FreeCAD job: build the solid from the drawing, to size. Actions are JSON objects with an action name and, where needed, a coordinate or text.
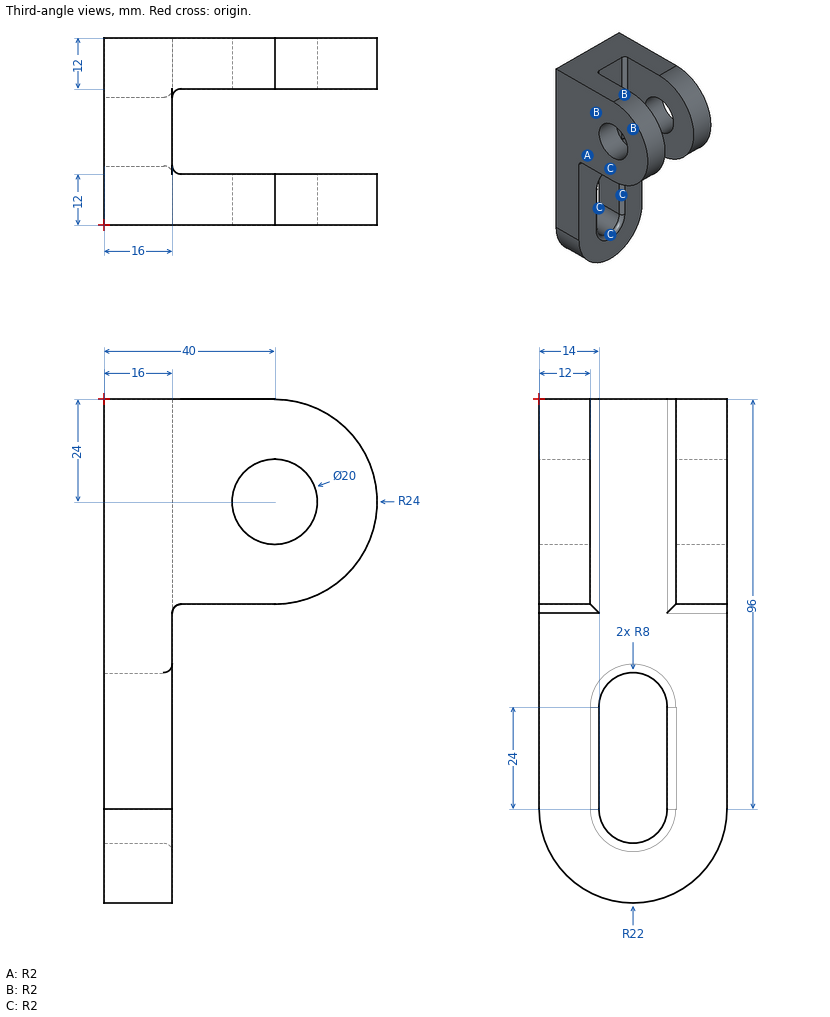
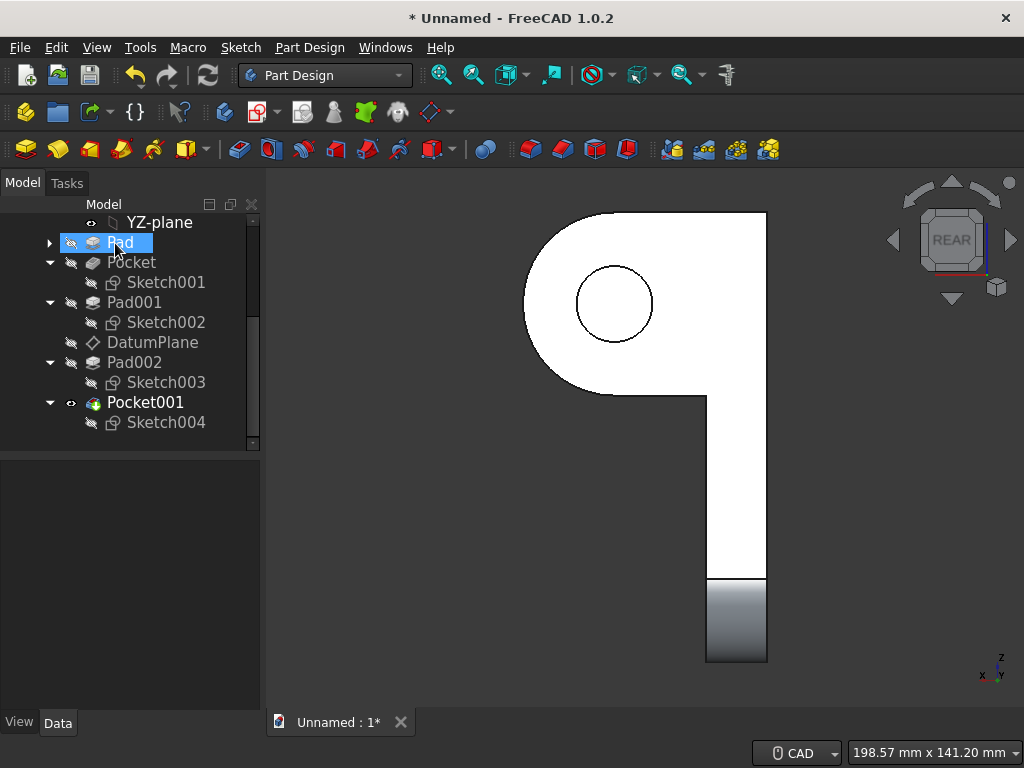
{"action": "left_click", "coordinate": [614, 303]}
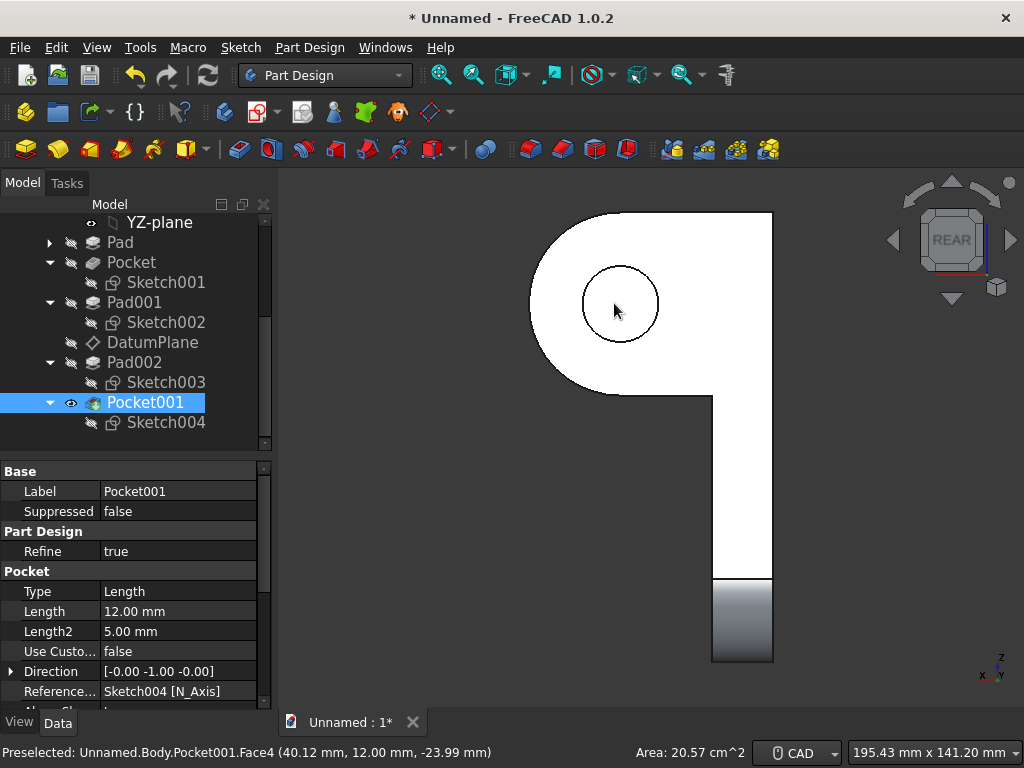
{"action": "left_click", "coordinate": [258, 112]}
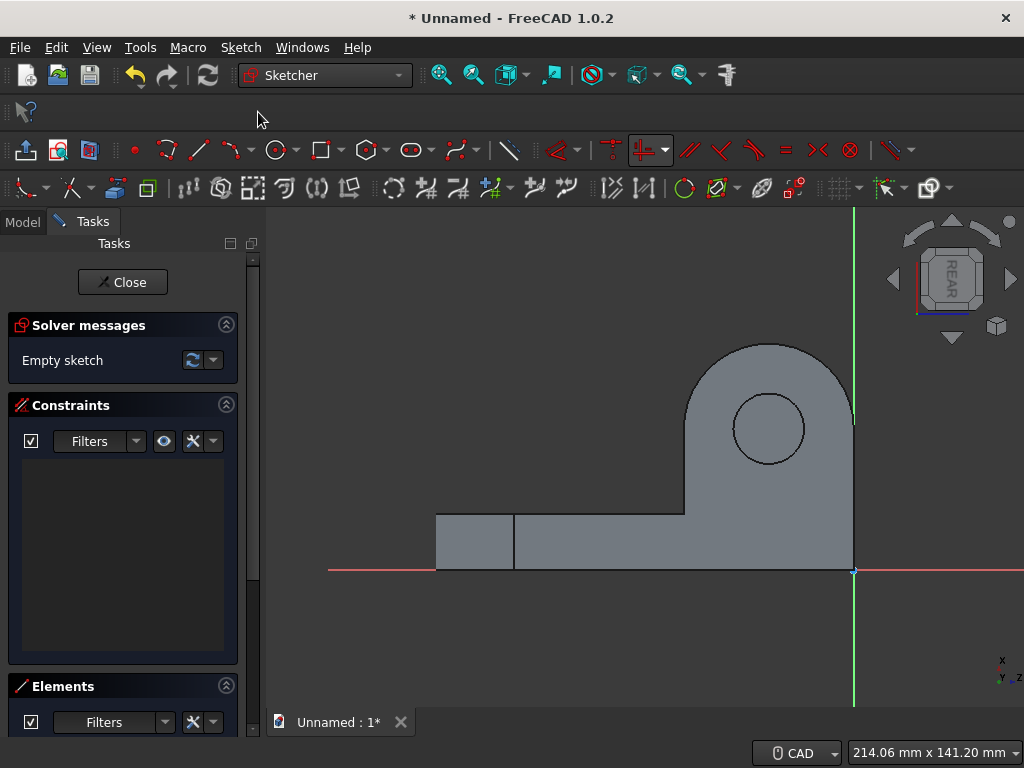
{"action": "scroll", "coordinate": [832, 419], "scroll_direction": "up", "scroll_amount": 7}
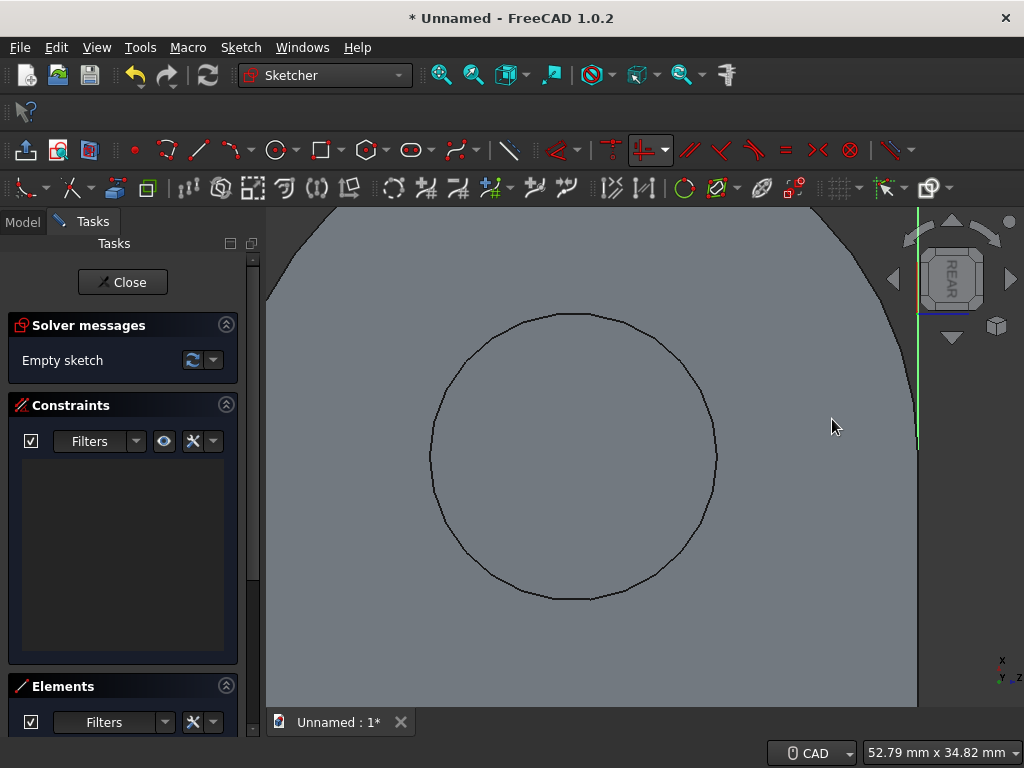
{"action": "left_click", "coordinate": [276, 150]}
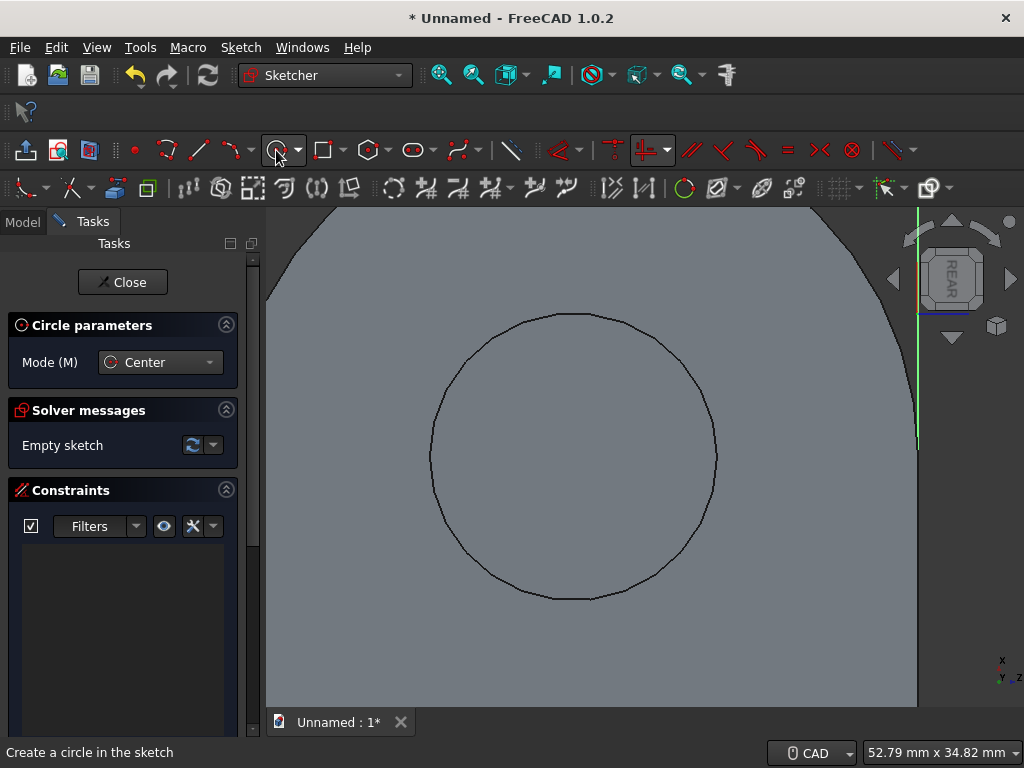
{"action": "left_click", "coordinate": [573, 457]}
{"action": "mouse_move", "coordinate": [675, 355]}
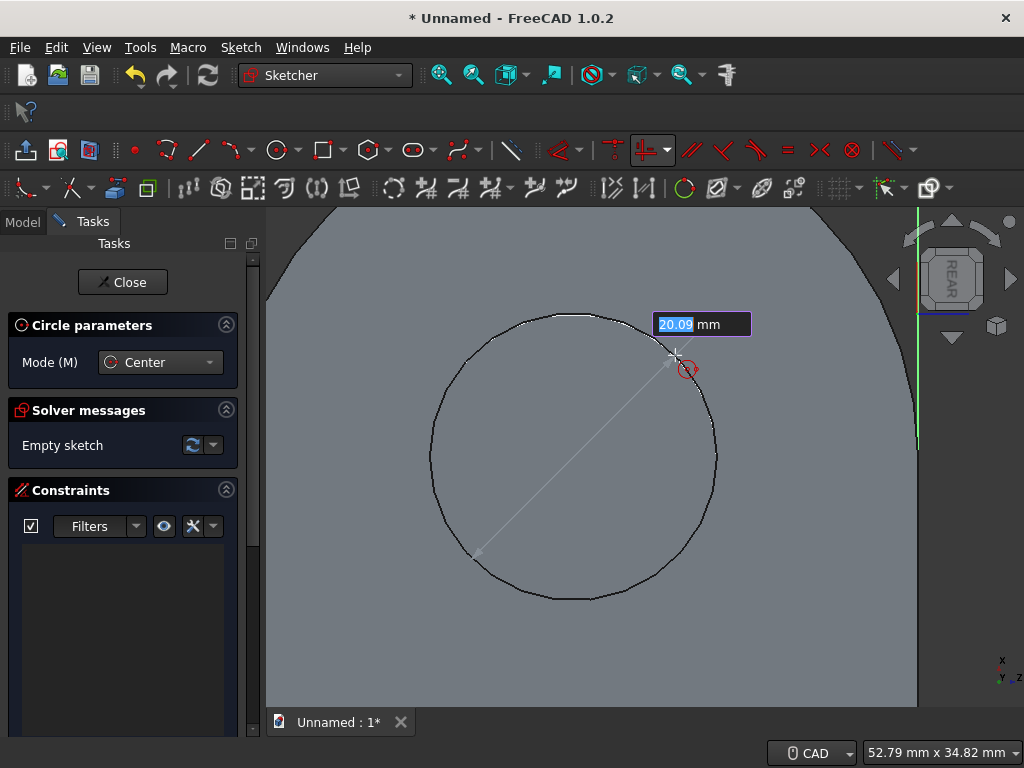
{"action": "type", "text": "20"}
{"action": "key", "text": "Return"}
{"action": "key", "text": "Escape"}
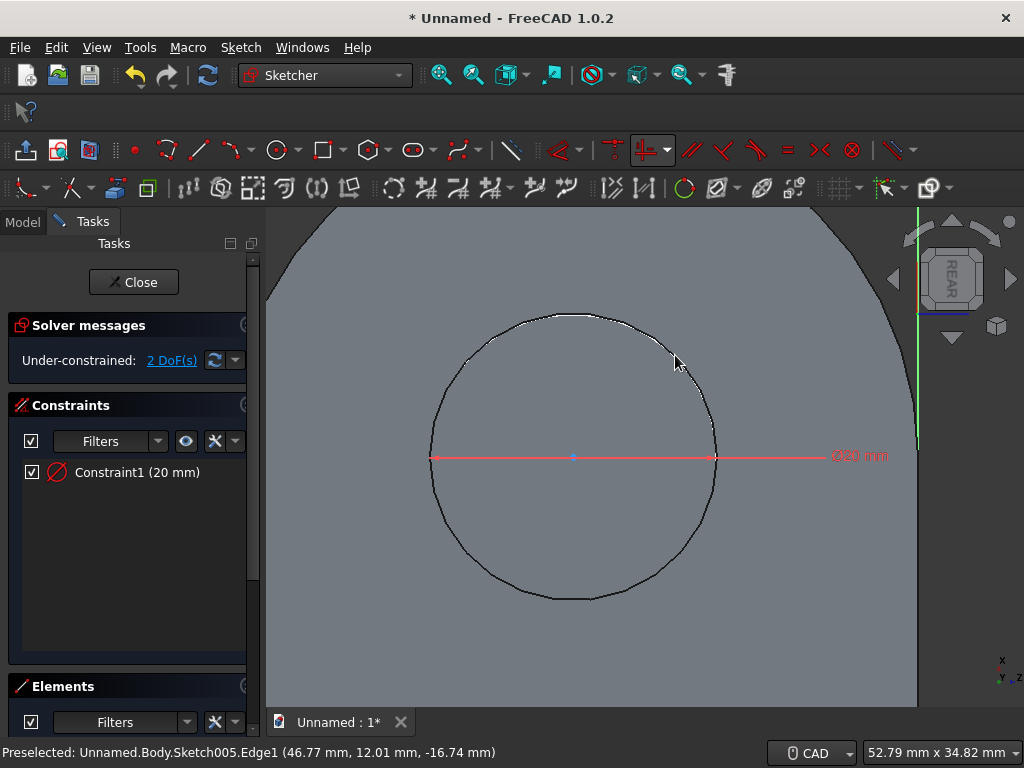
{"action": "left_click", "coordinate": [558, 150]}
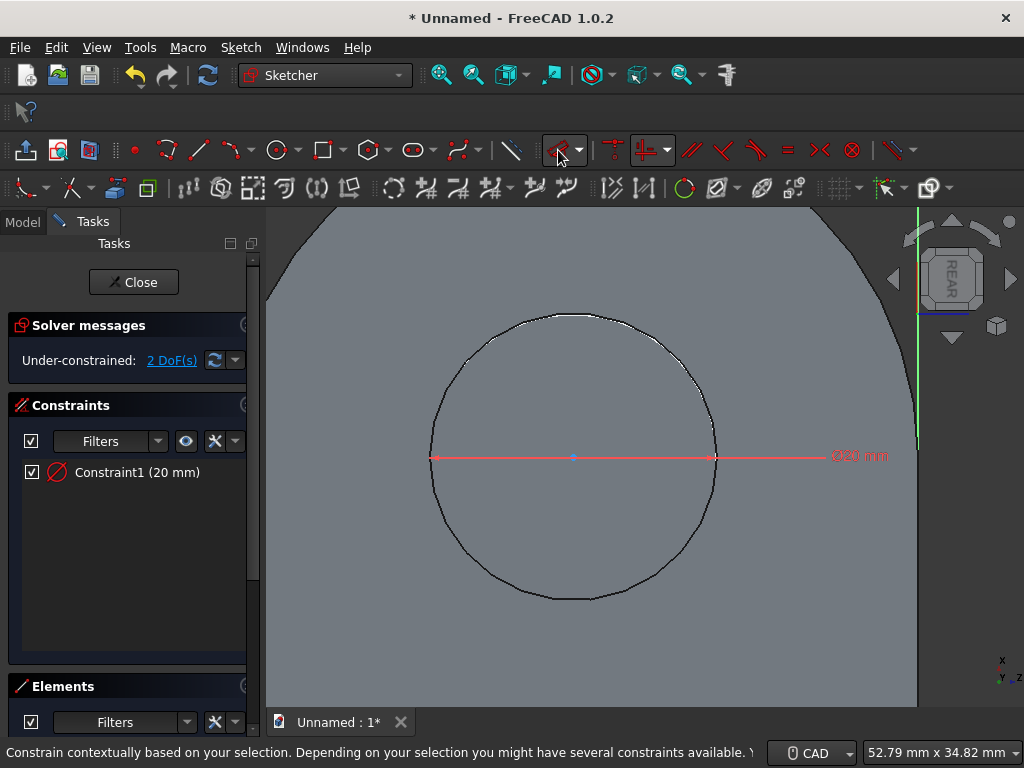
{"action": "left_click", "coordinate": [573, 458]}
{"action": "left_click", "coordinate": [650, 424]}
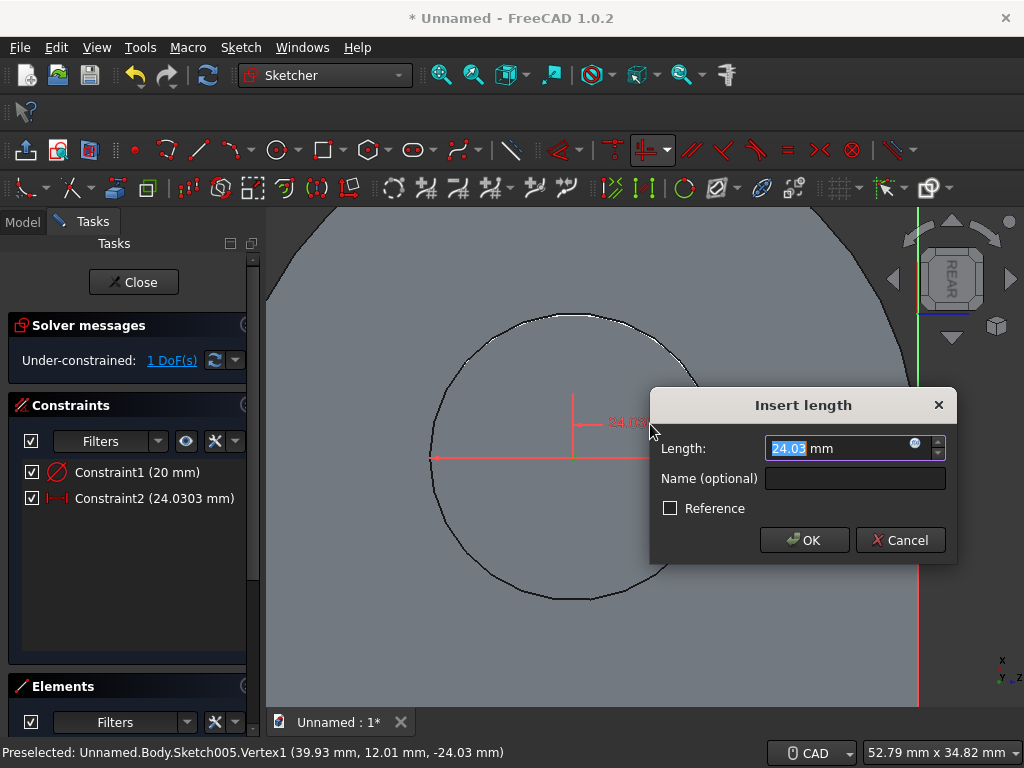
{"action": "type", "text": "24"}
{"action": "key", "text": "Return"}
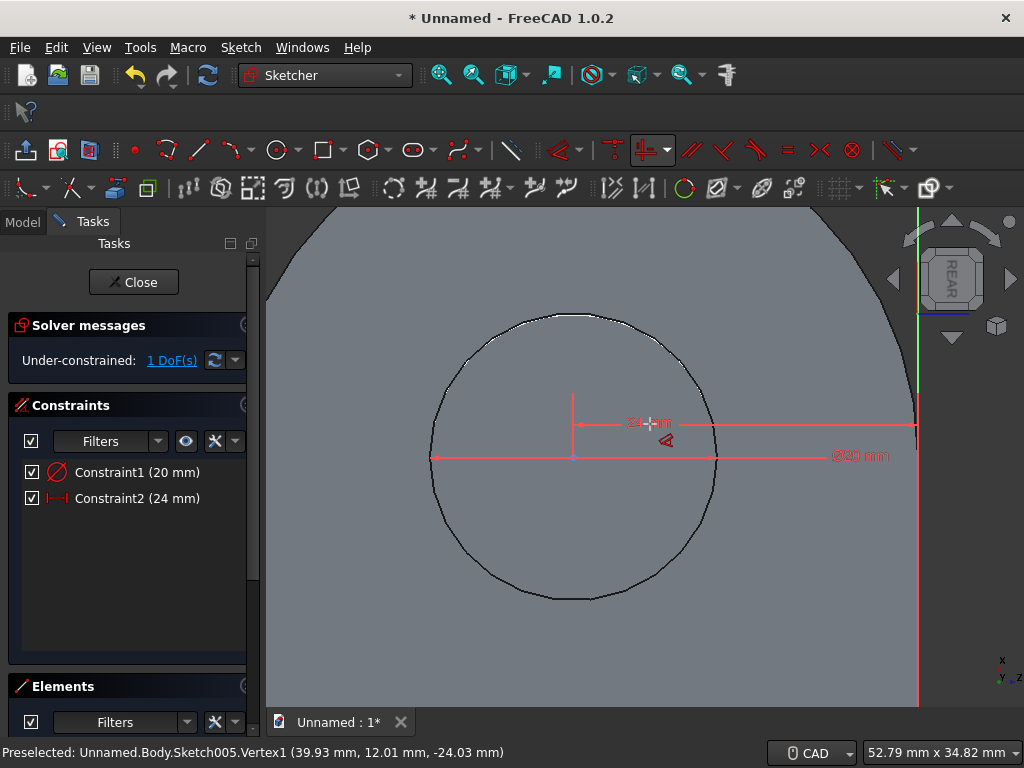
{"action": "left_click", "coordinate": [573, 458]}
{"action": "left_click", "coordinate": [539, 569]}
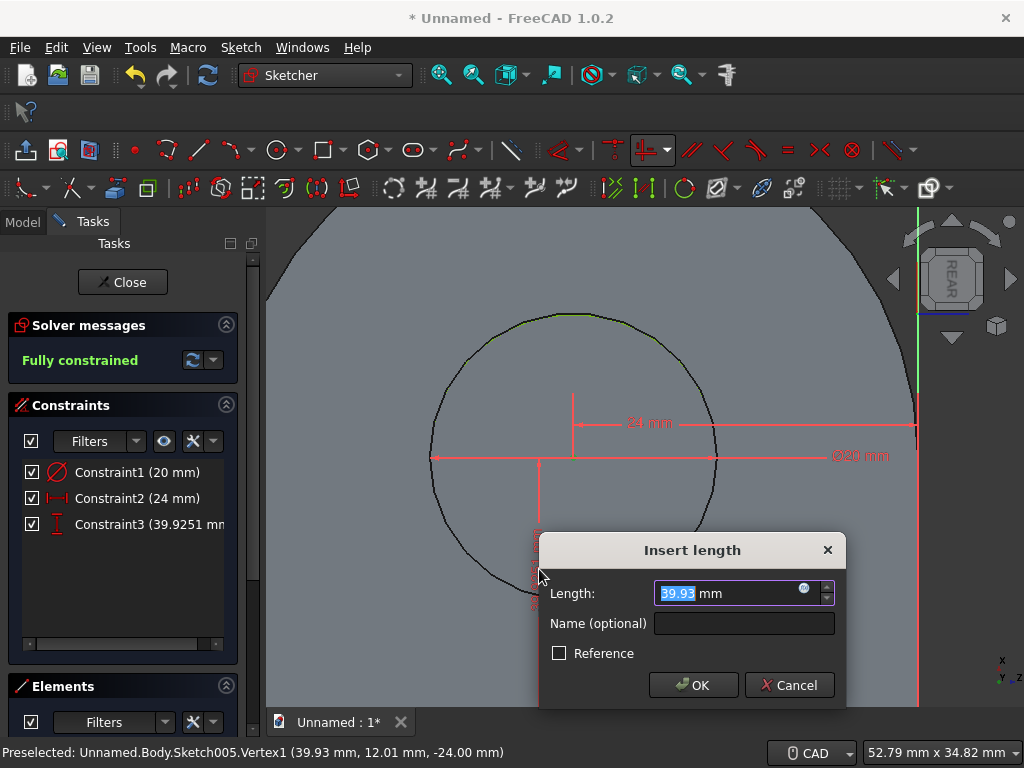
{"action": "type", "text": "40"}
{"action": "key", "text": "Return"}
{"action": "key", "text": "Escape"}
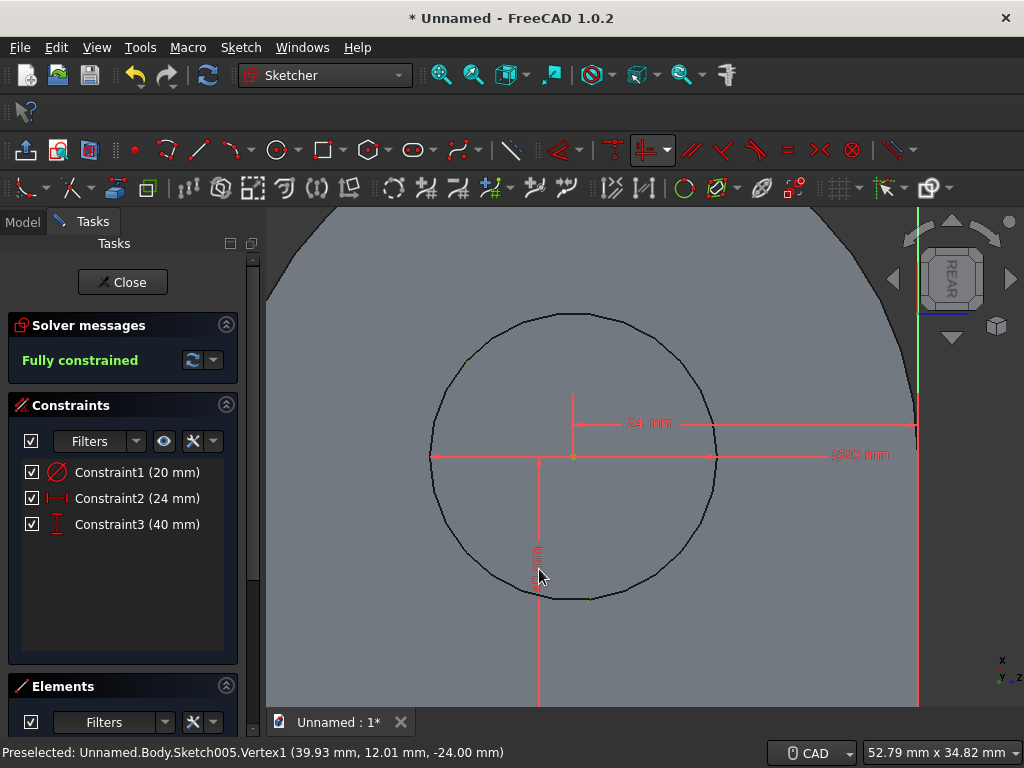
{"action": "left_click", "coordinate": [123, 282]}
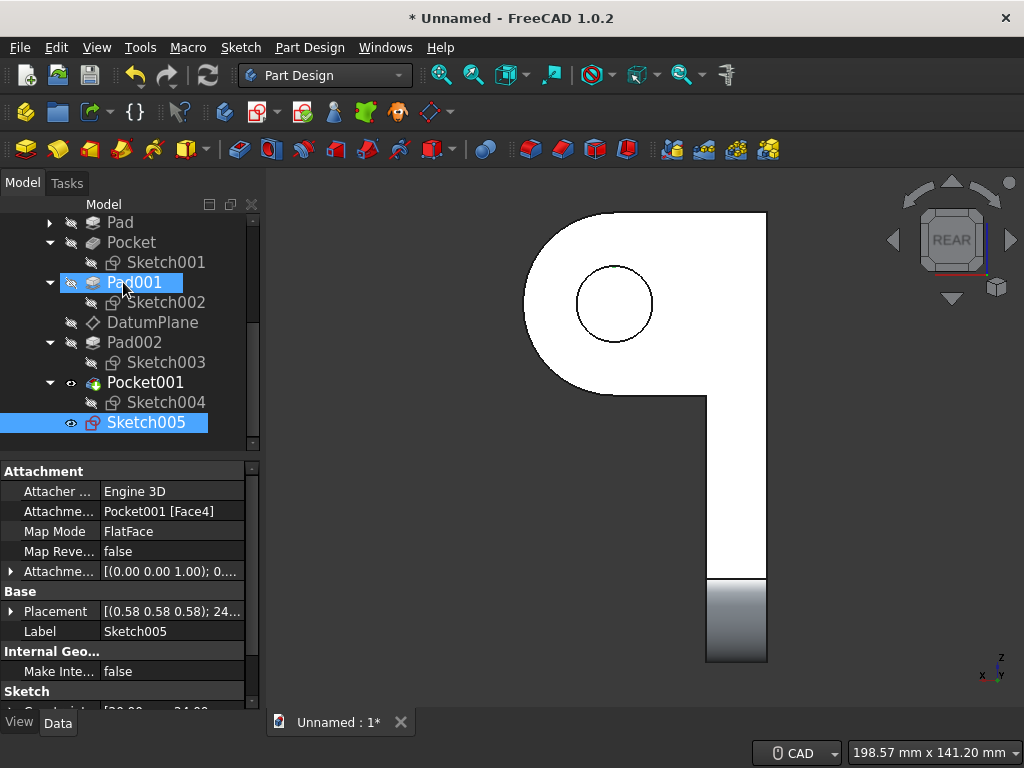
{"action": "left_click", "coordinate": [240, 150]}